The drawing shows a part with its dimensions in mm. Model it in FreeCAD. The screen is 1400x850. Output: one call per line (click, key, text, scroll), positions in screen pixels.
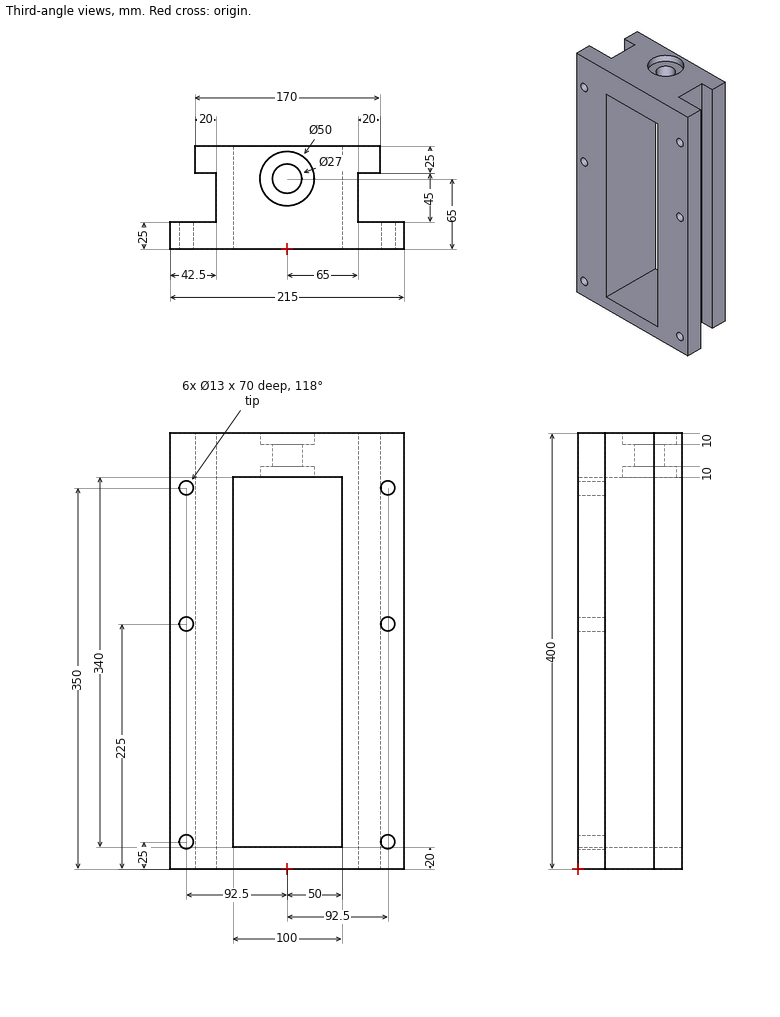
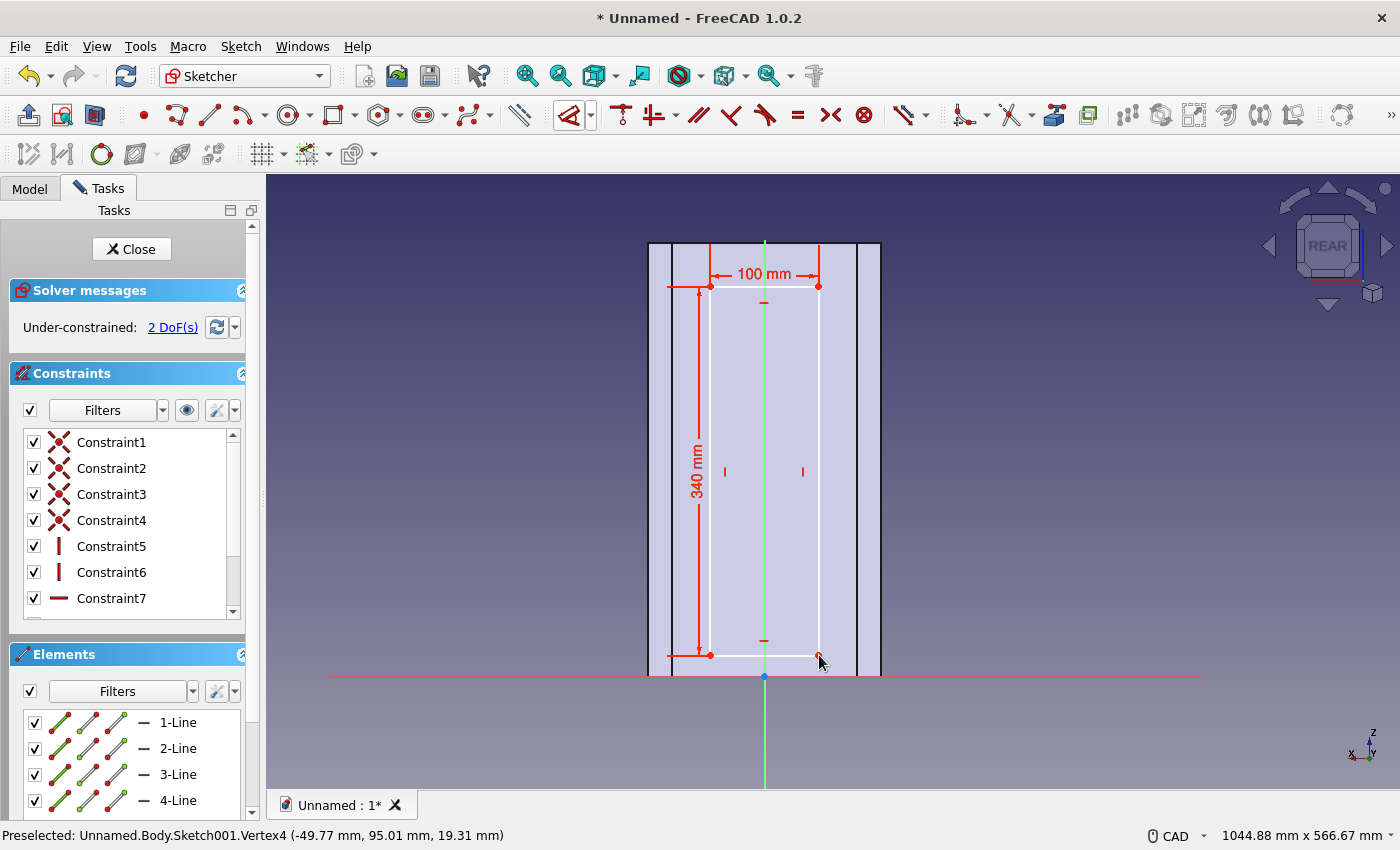
click(710, 287)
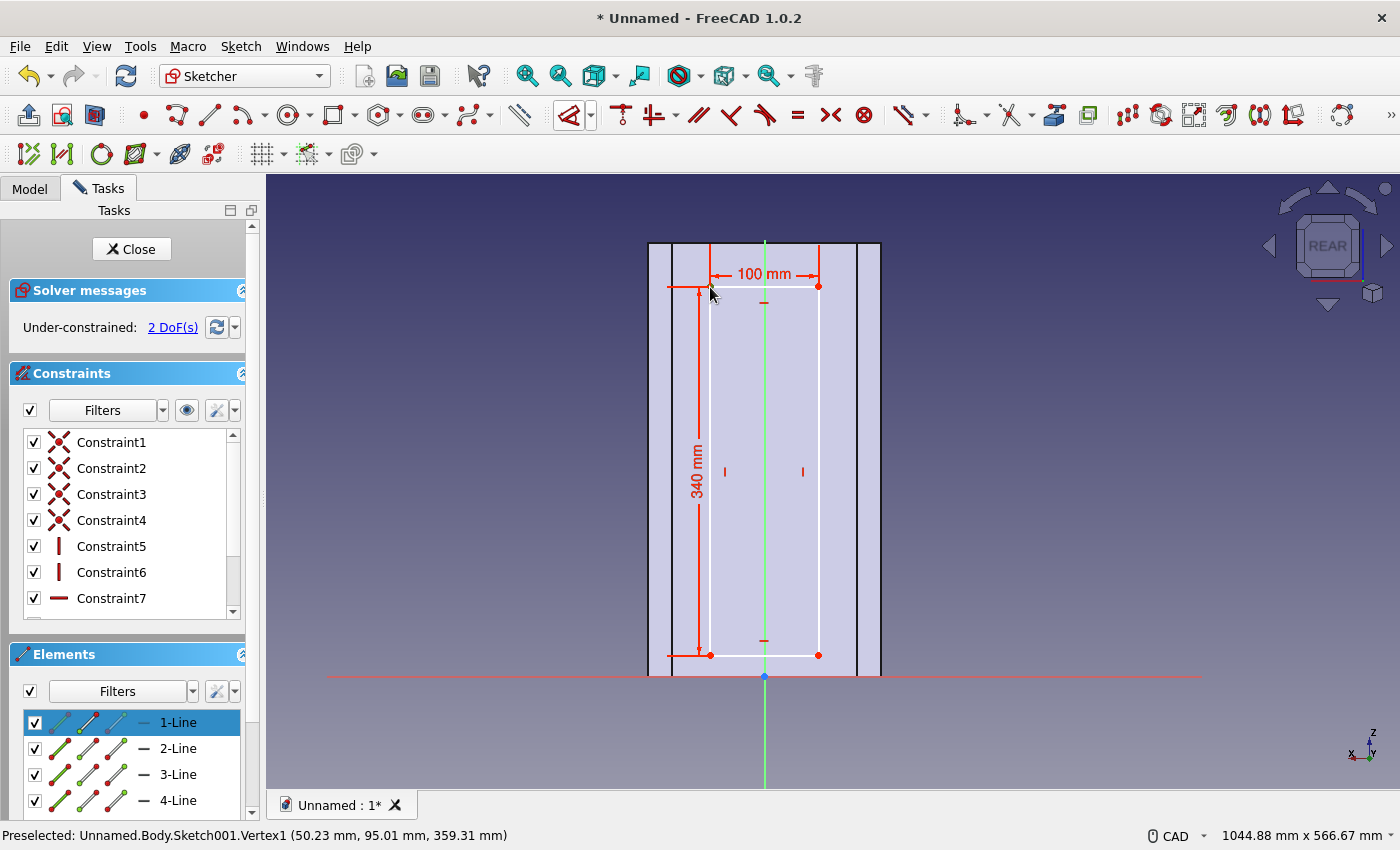
key(l)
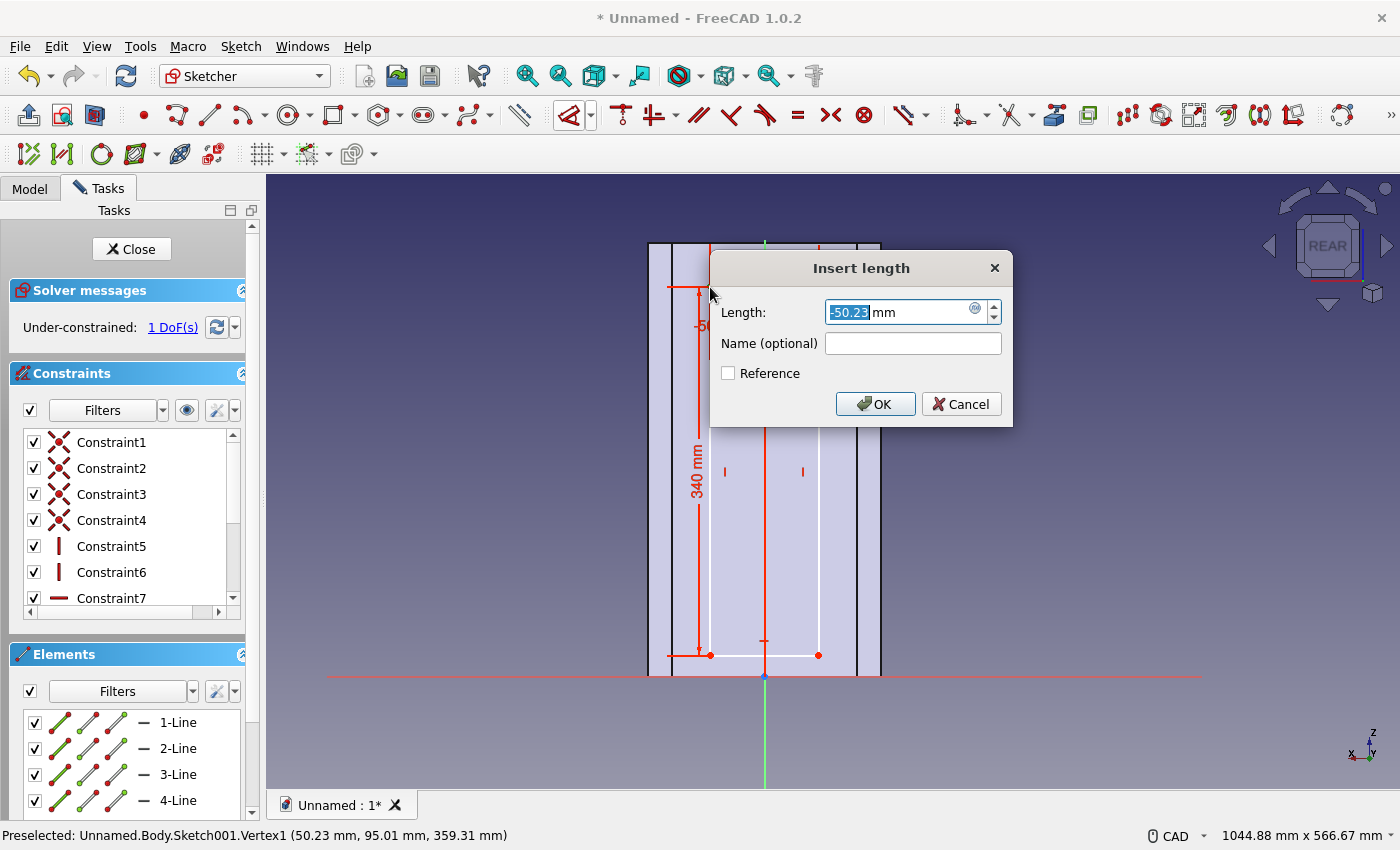
text(-50)
key(Return)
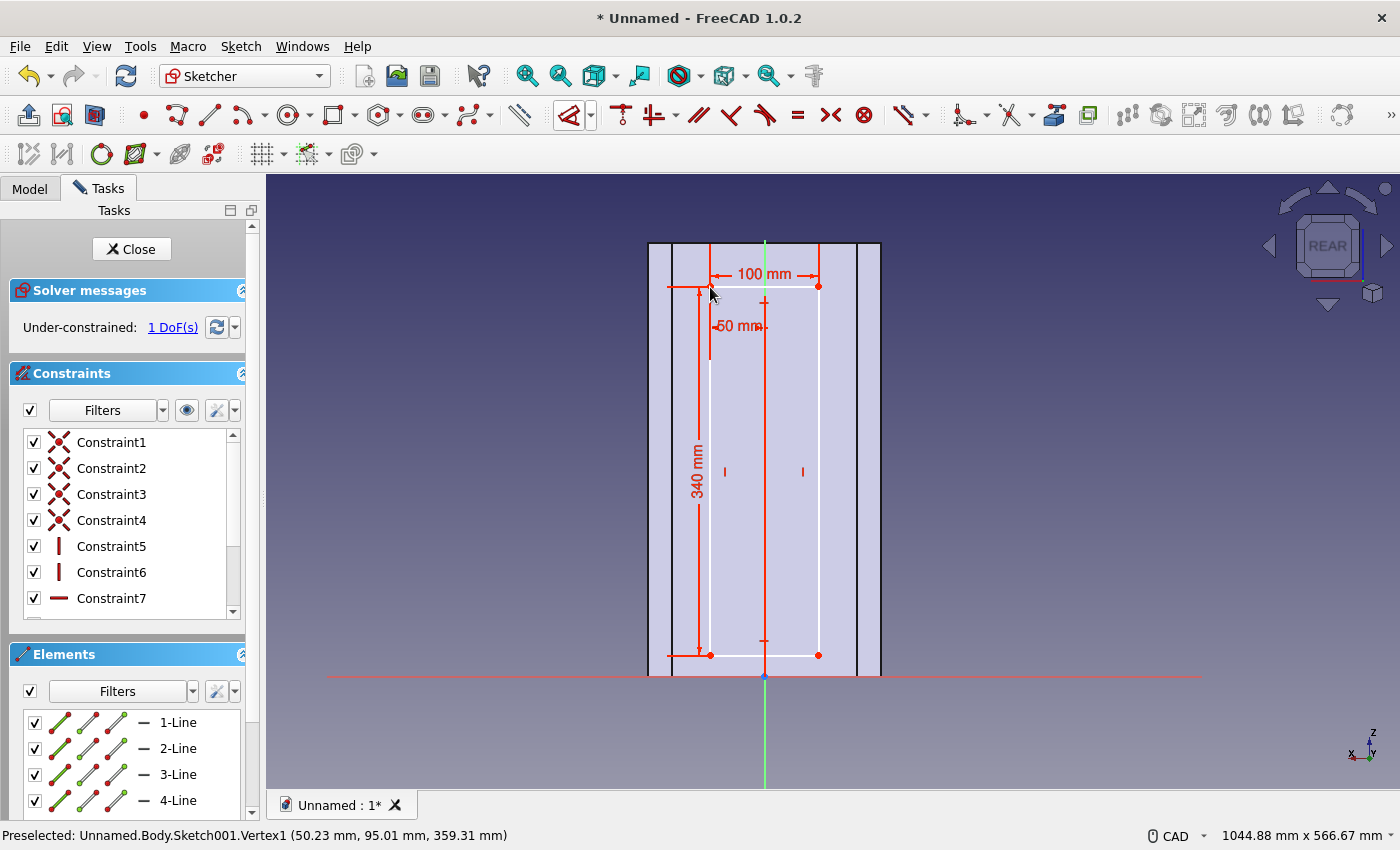
scroll(710, 656, up, 4)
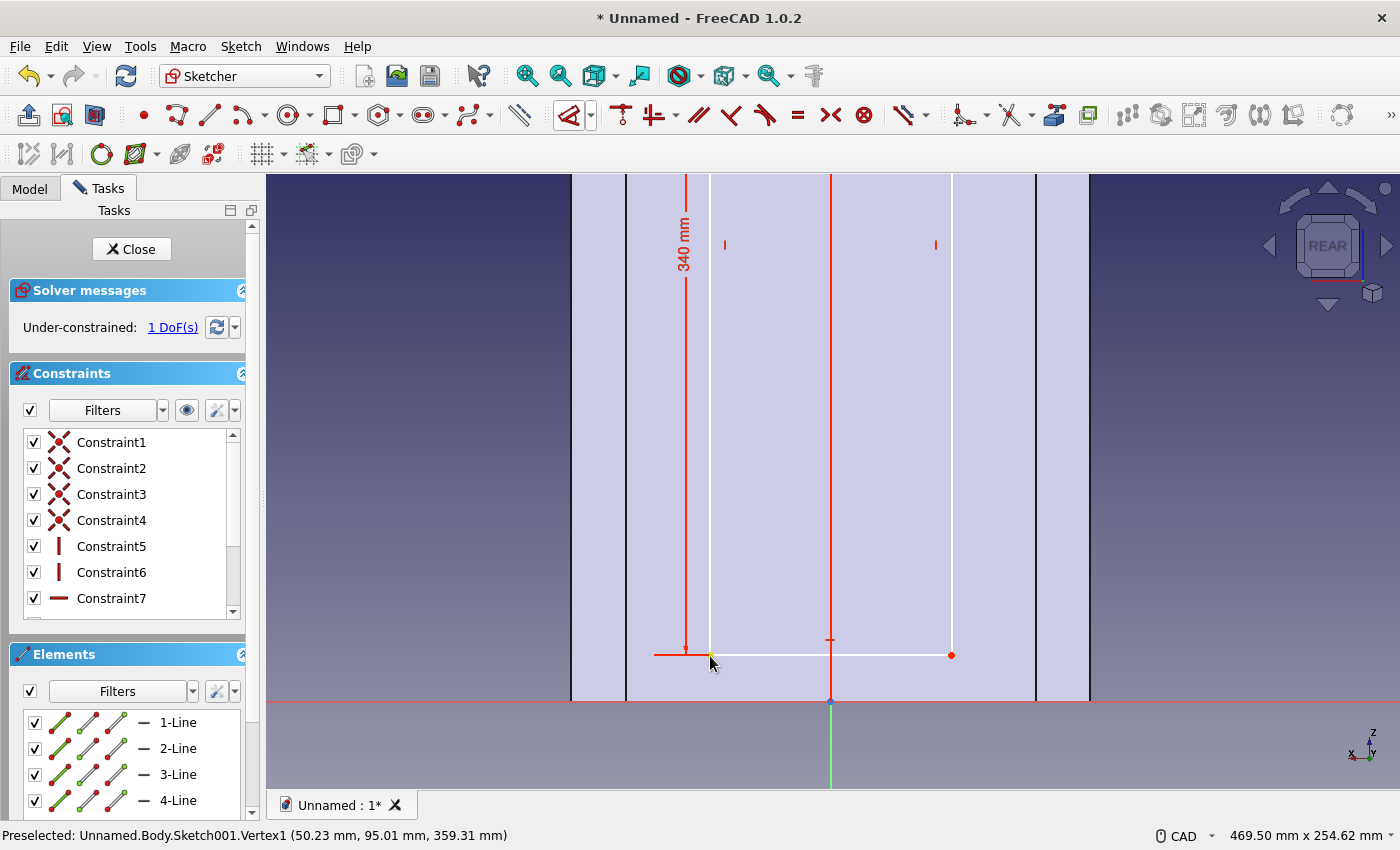
click(710, 655)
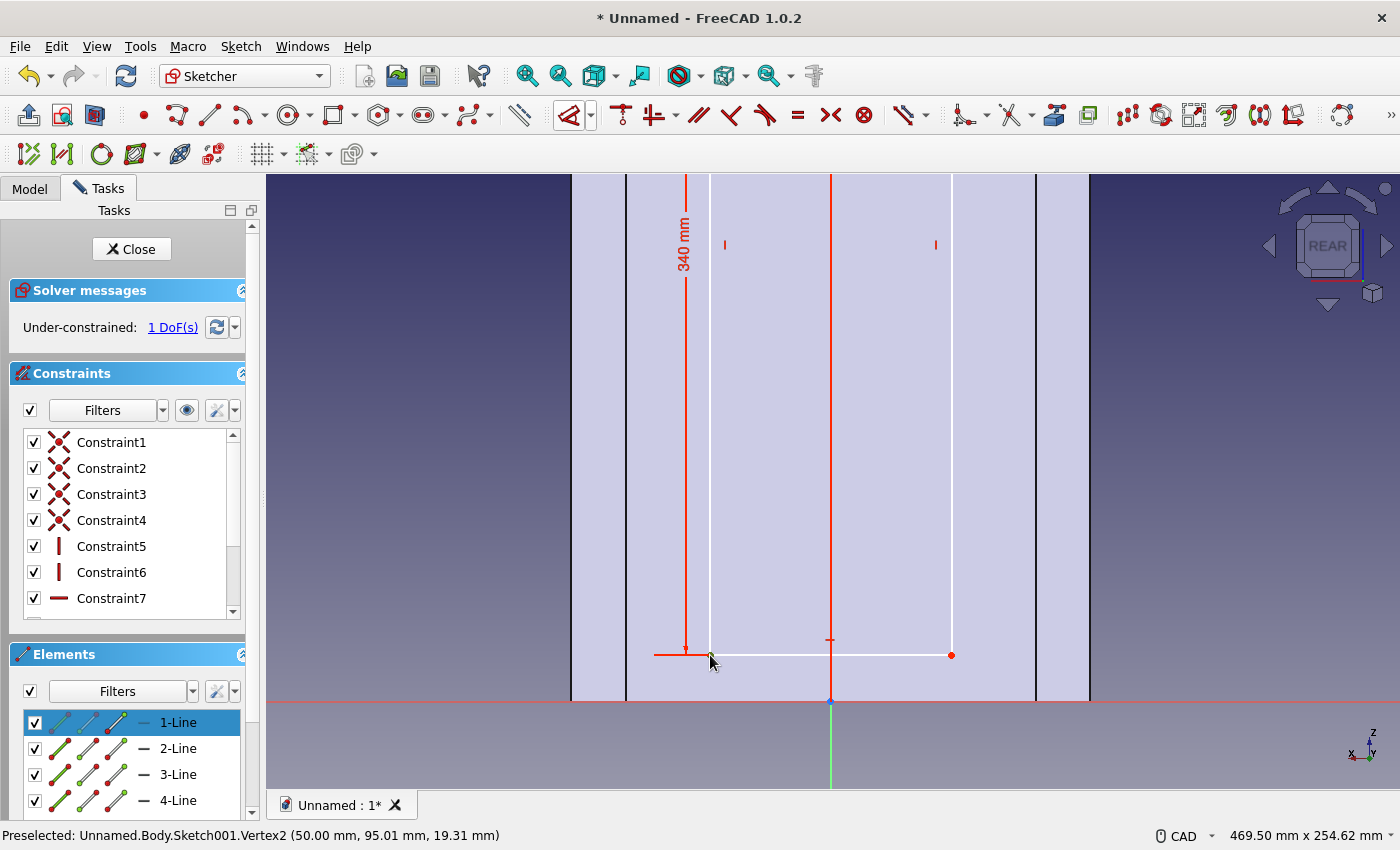
key(i)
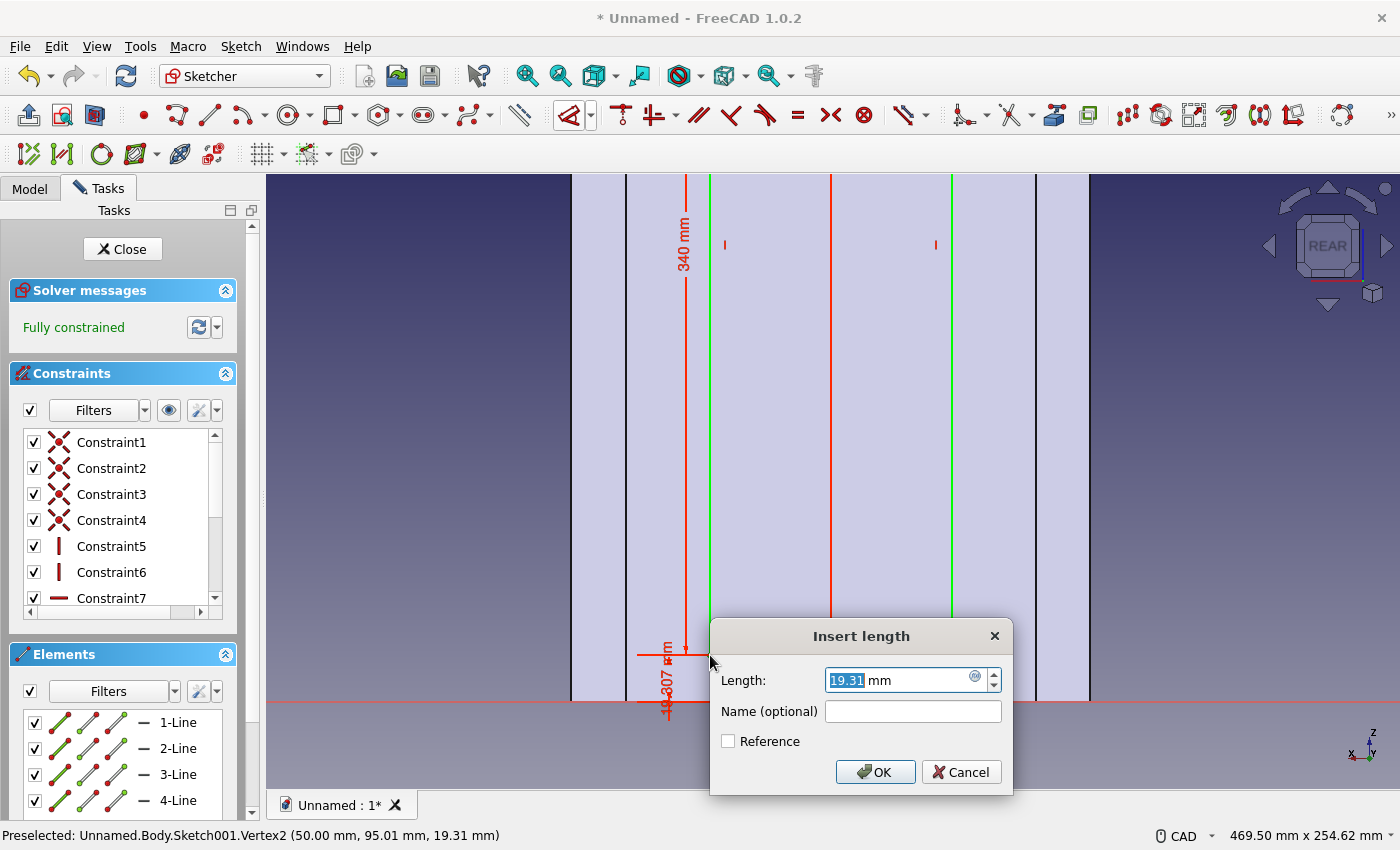
text(20)
key(Return)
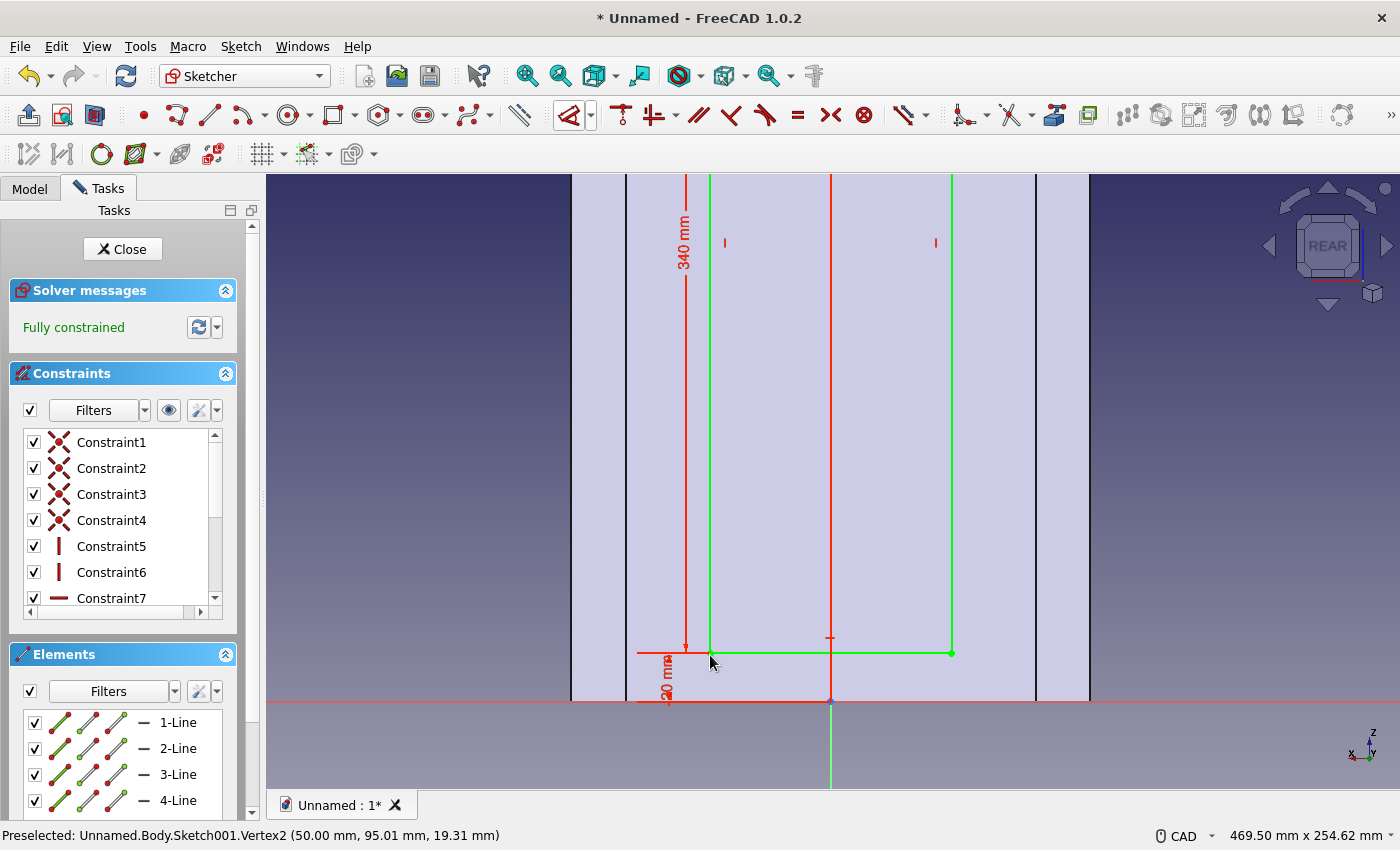
click(123, 249)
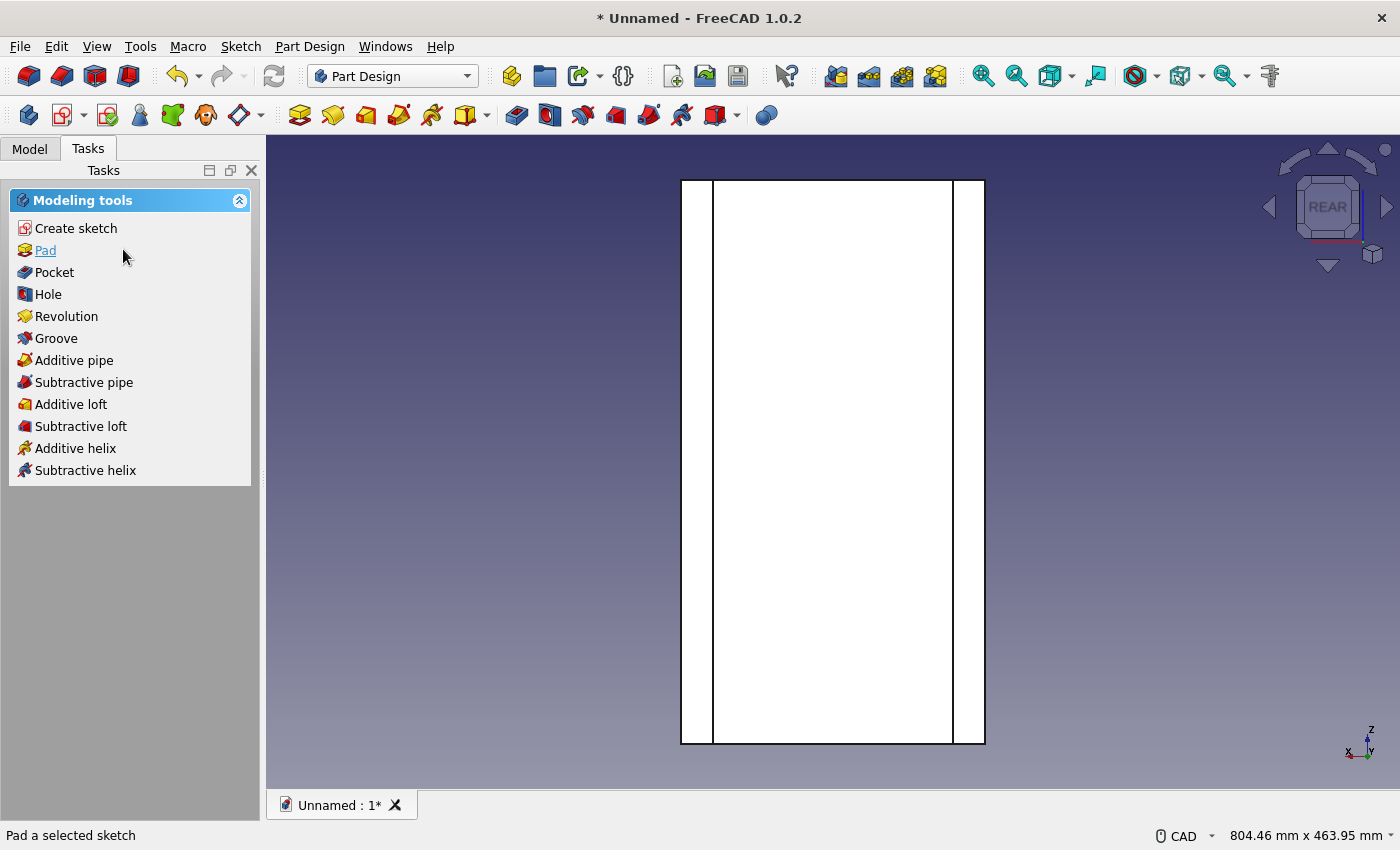
click(517, 116)